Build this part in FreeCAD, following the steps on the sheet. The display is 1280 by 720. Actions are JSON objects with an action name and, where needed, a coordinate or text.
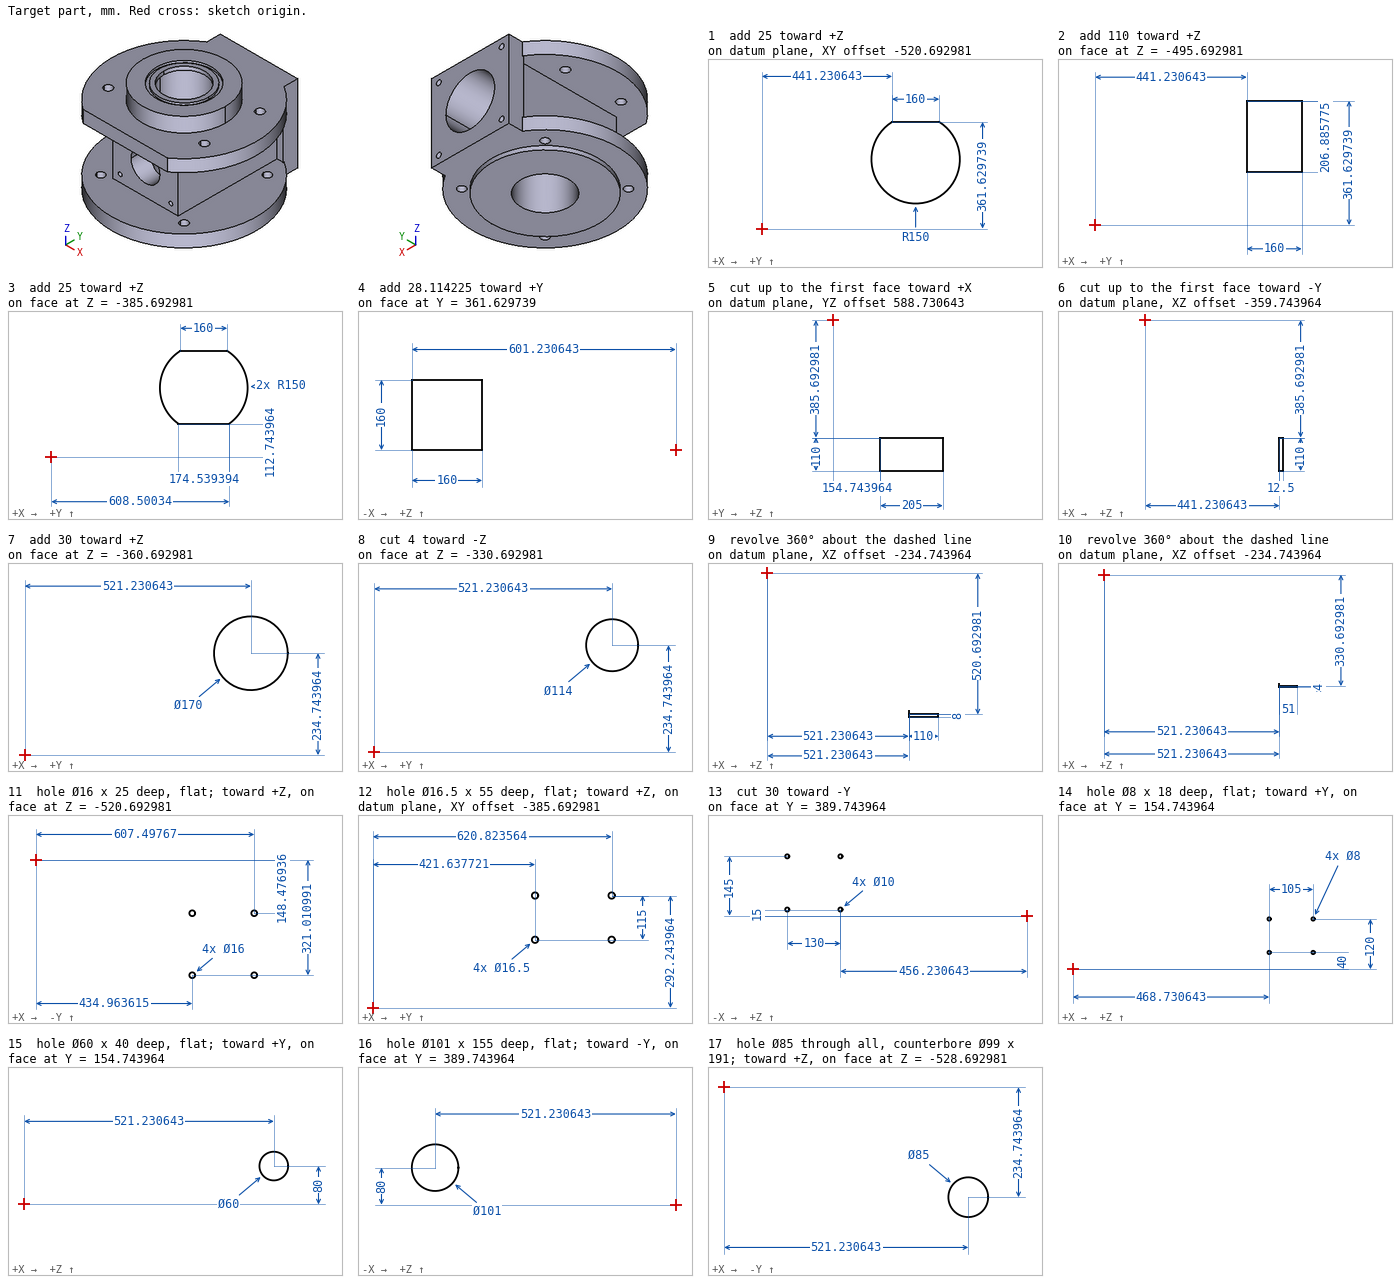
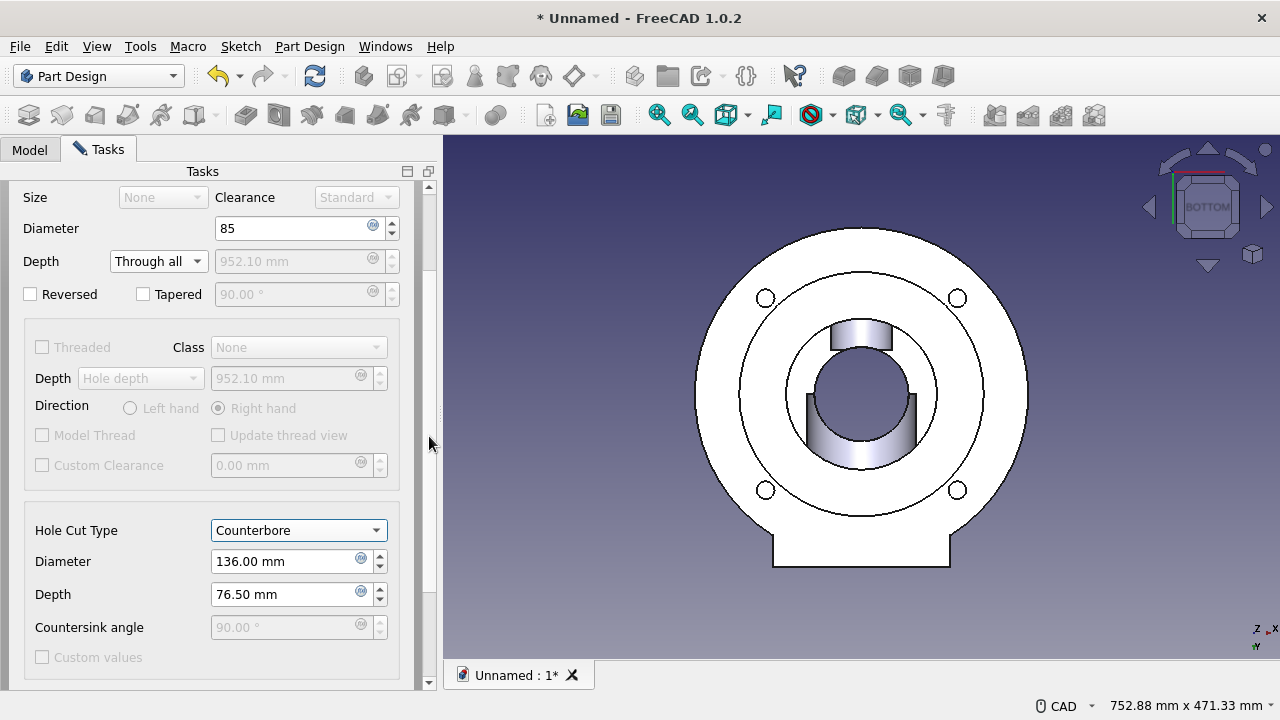
{"action": "triple_click", "coordinate": [292, 562]}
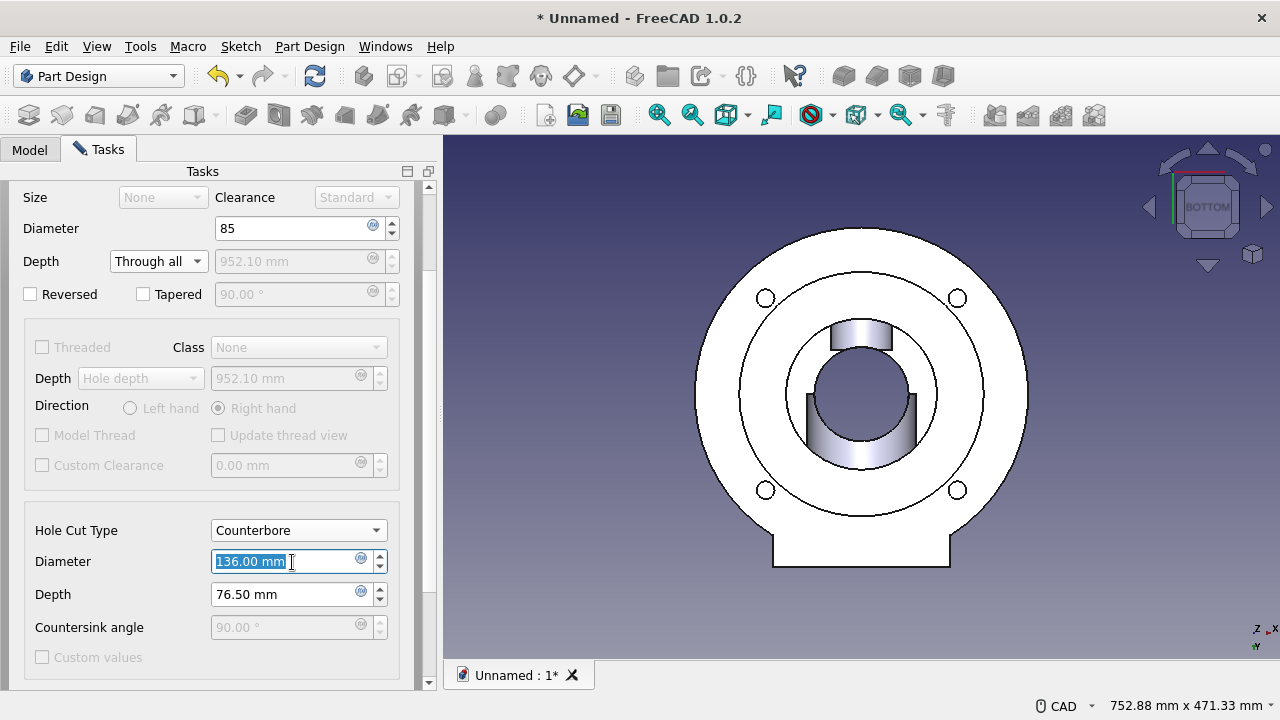
{"action": "type", "text": "99"}
{"action": "key", "text": "Tab"}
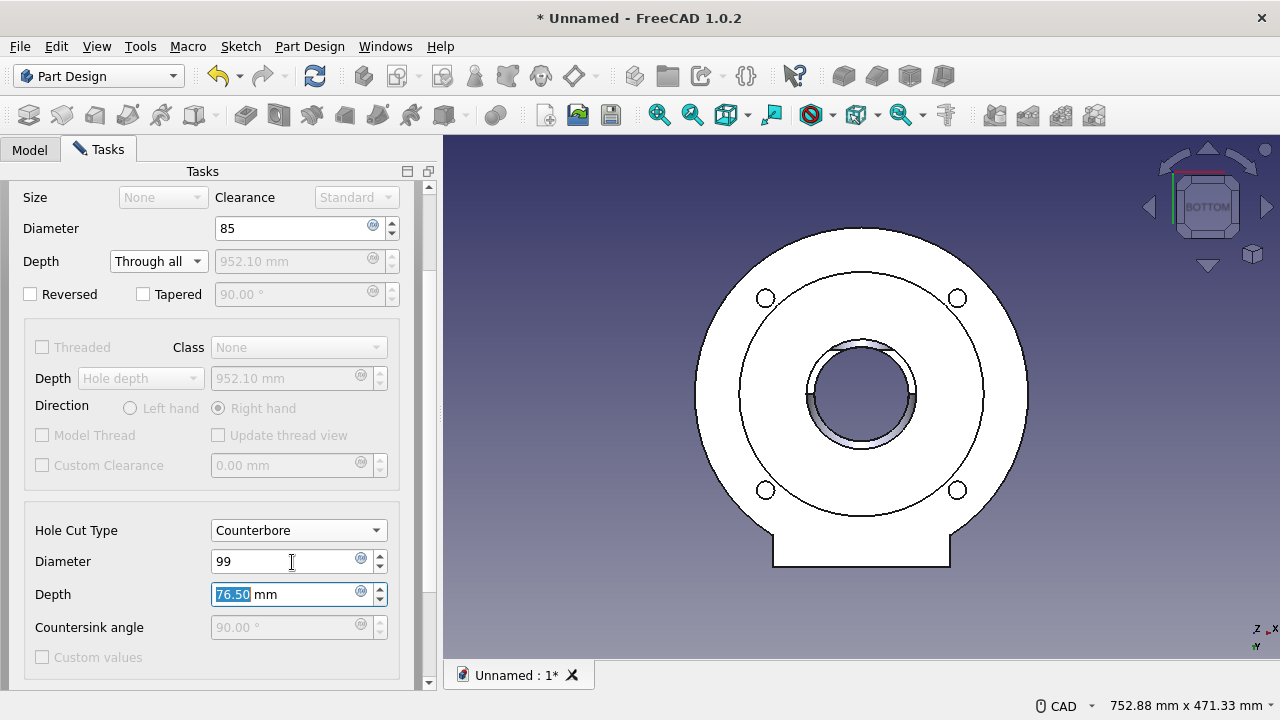
{"action": "type", "text": "191"}
{"action": "key", "text": "Tab"}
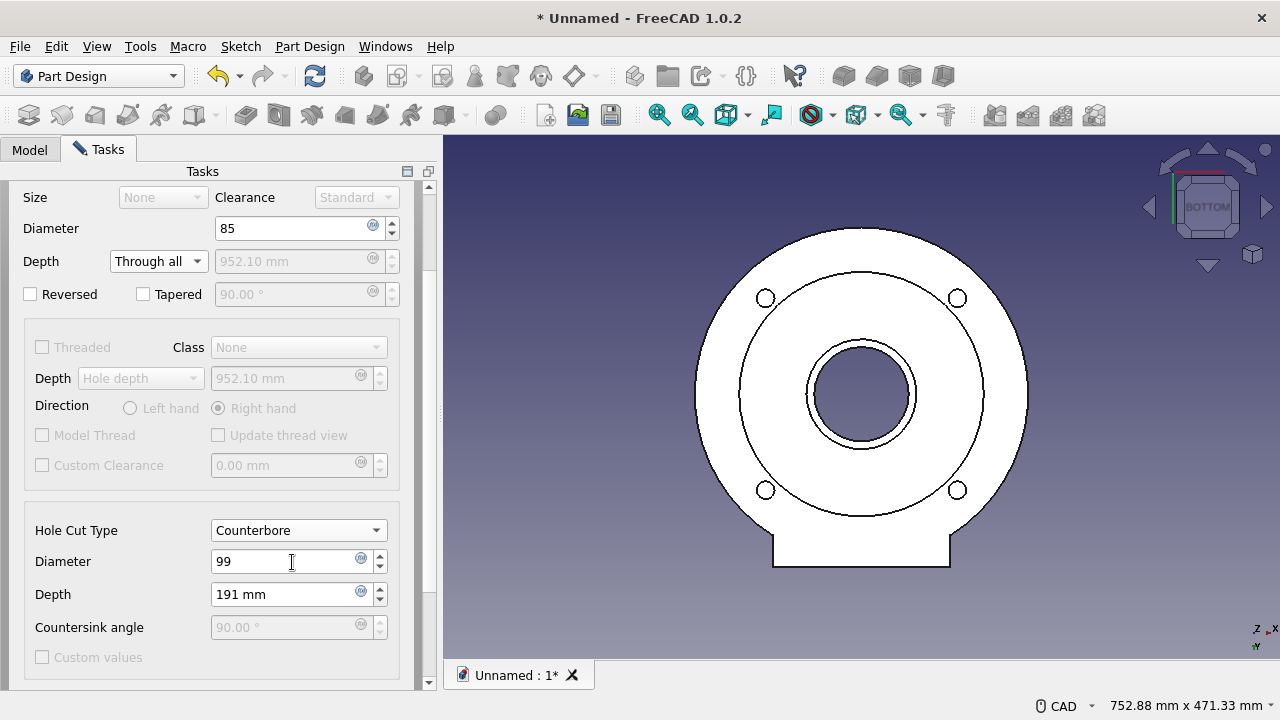
{"action": "scroll", "coordinate": [429, 436], "scroll_direction": "up", "scroll_amount": 3}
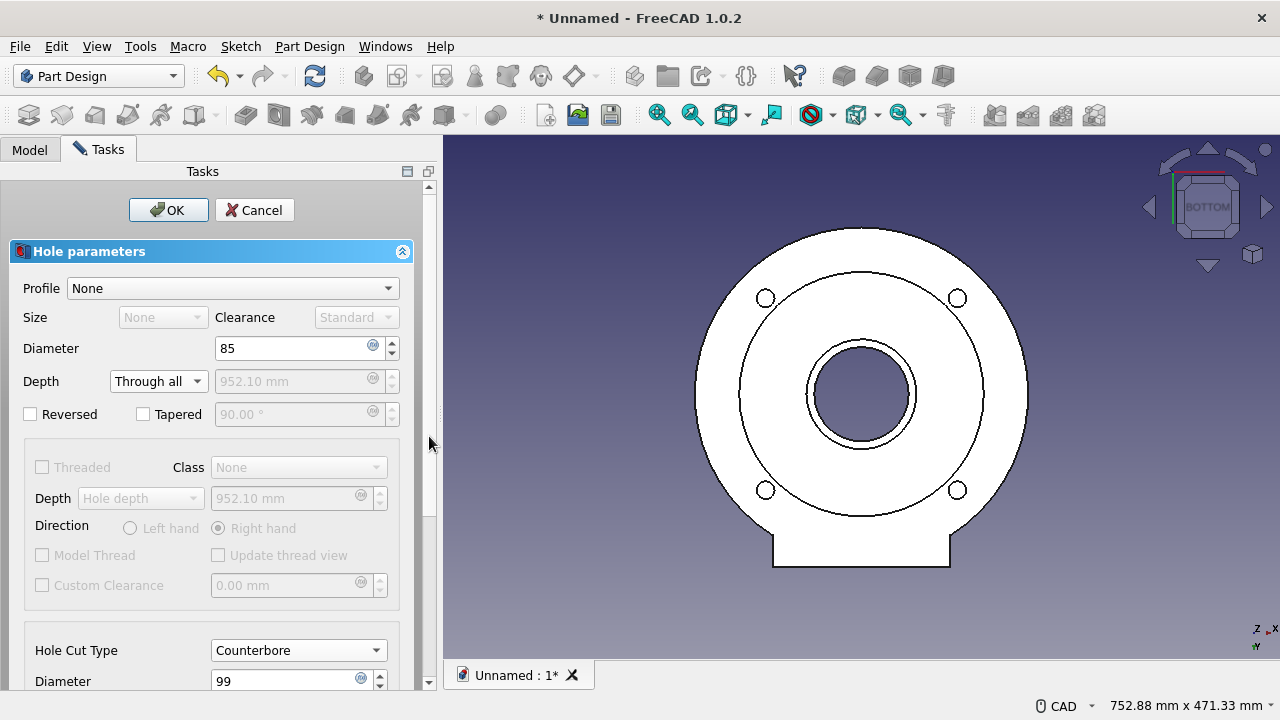
{"action": "left_click", "coordinate": [169, 210]}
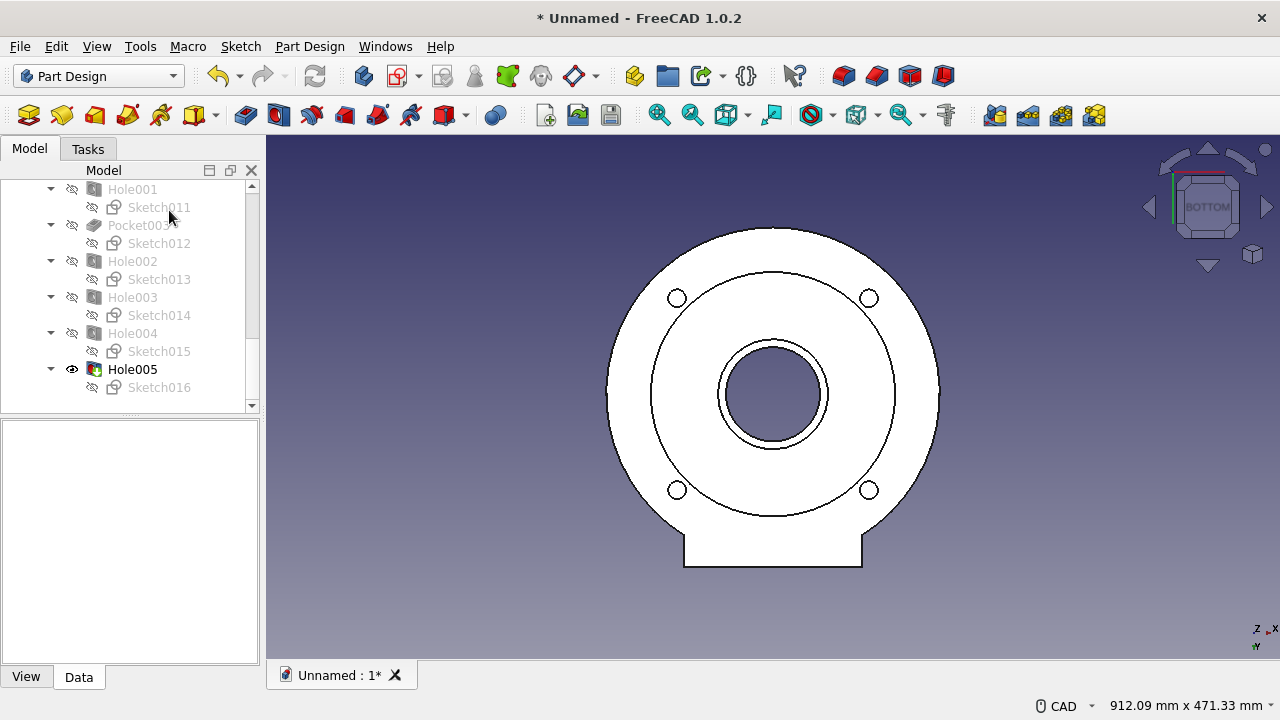
{"action": "key", "text": "0"}